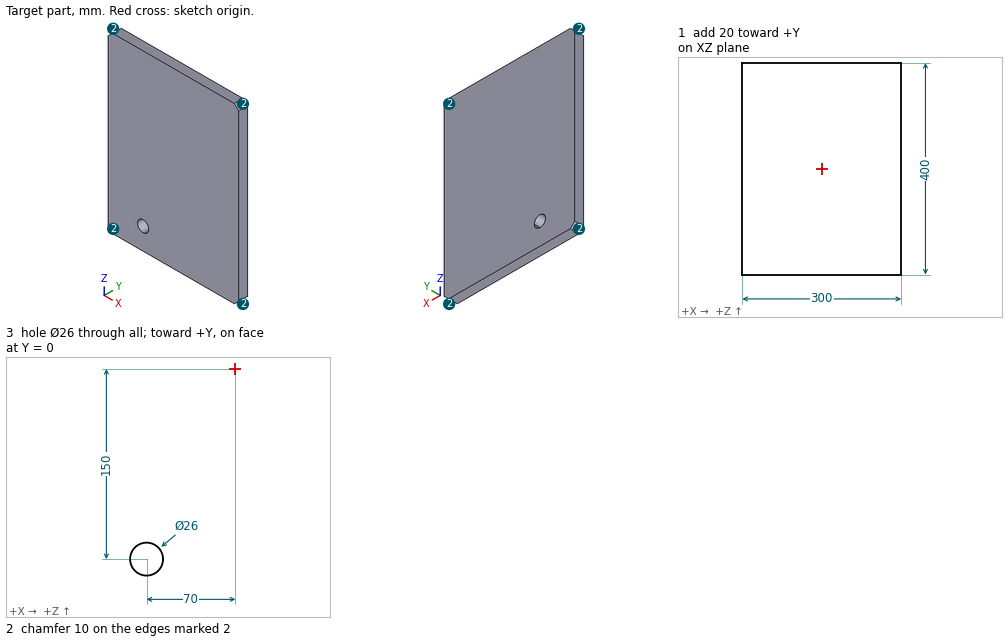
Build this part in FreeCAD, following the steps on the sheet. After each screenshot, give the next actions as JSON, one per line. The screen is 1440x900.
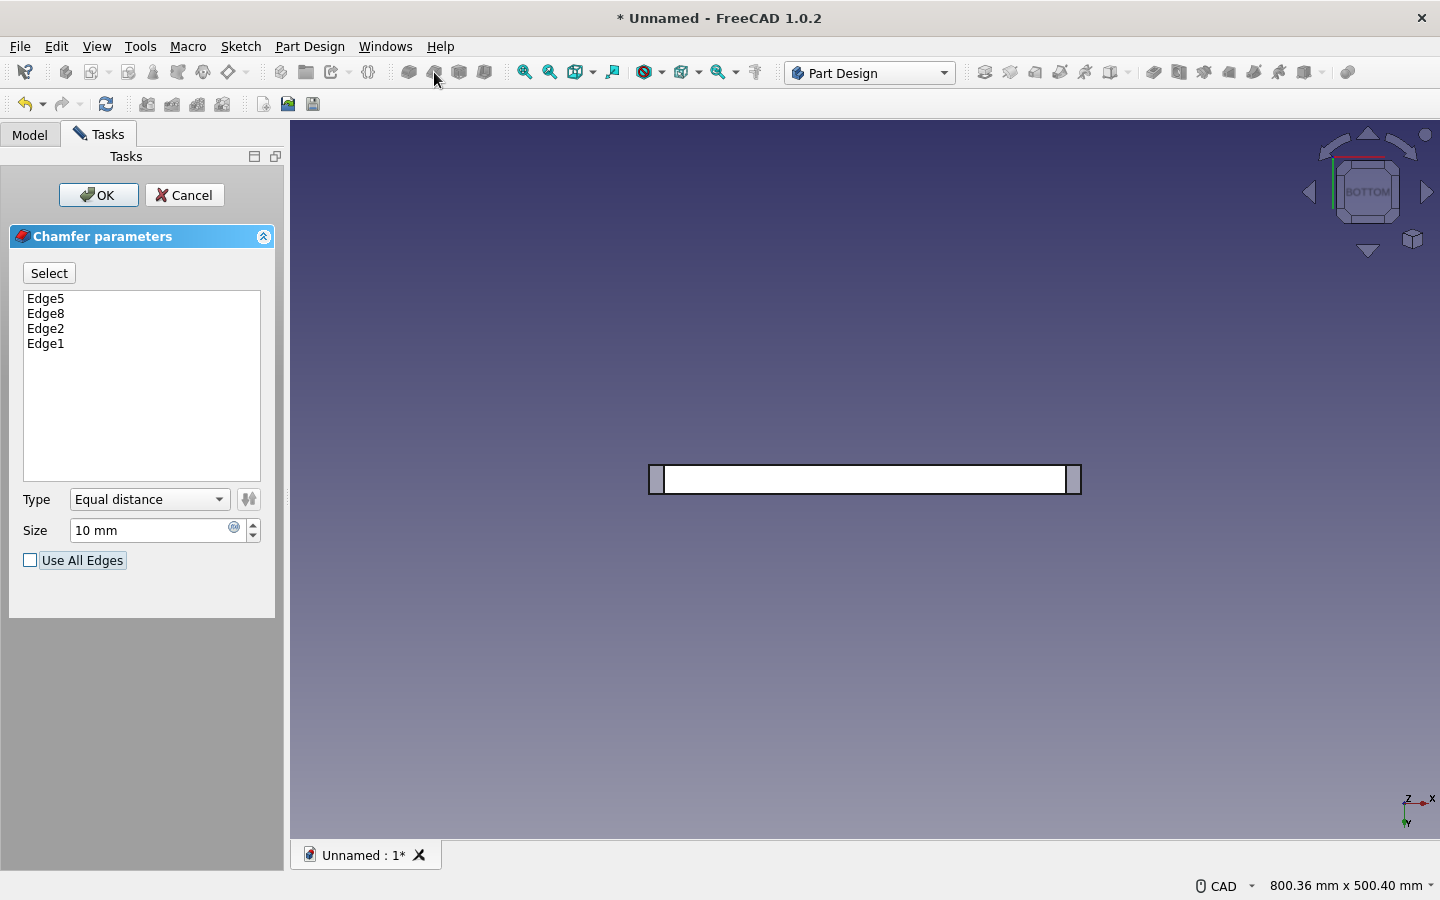
{"action": "left_click", "coordinate": [99, 195]}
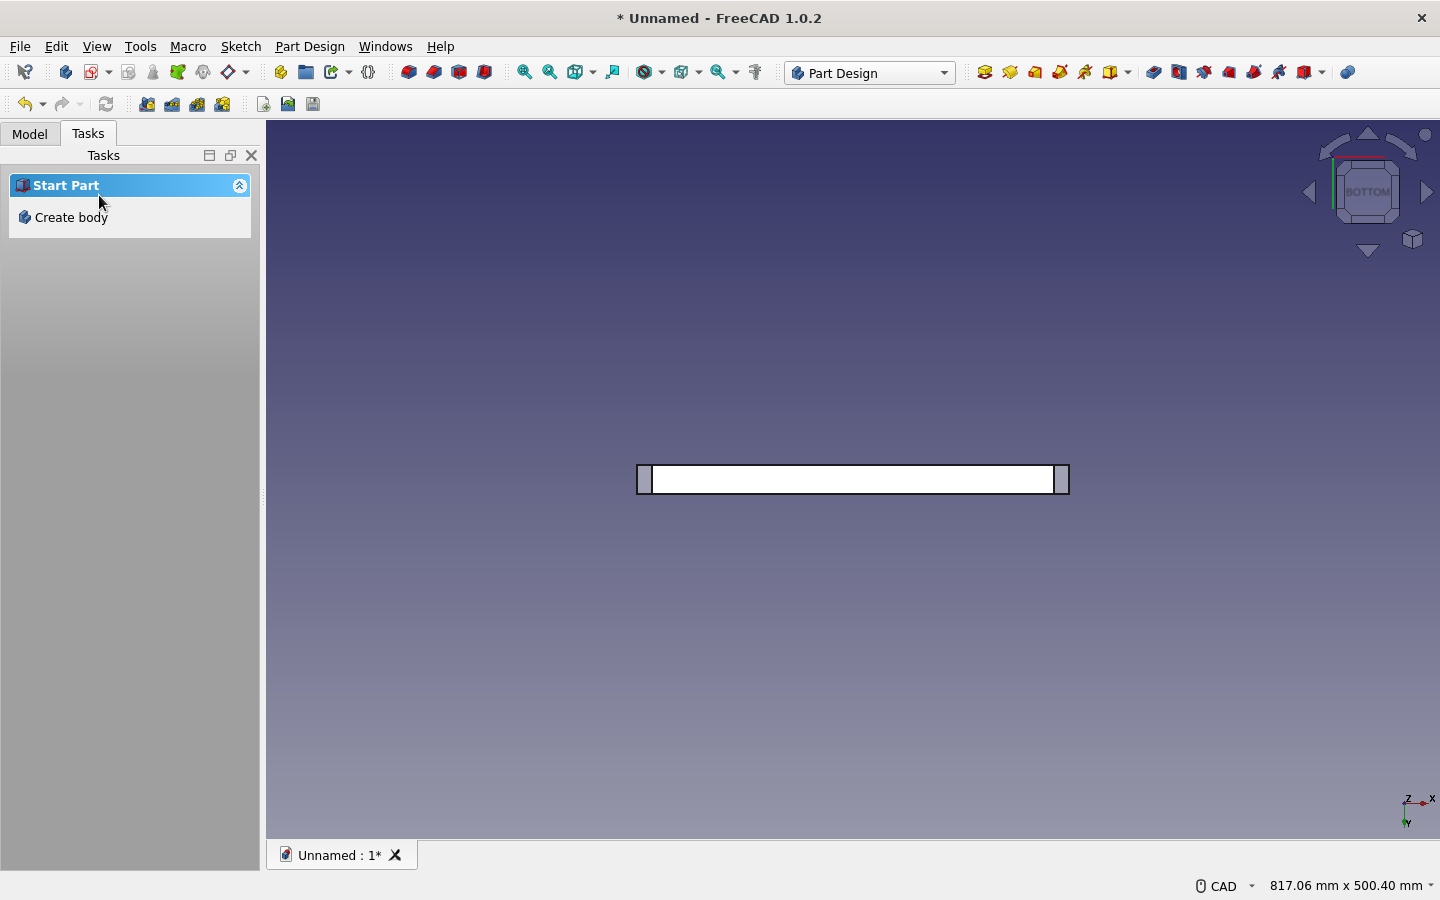
{"action": "left_click", "coordinate": [525, 72]}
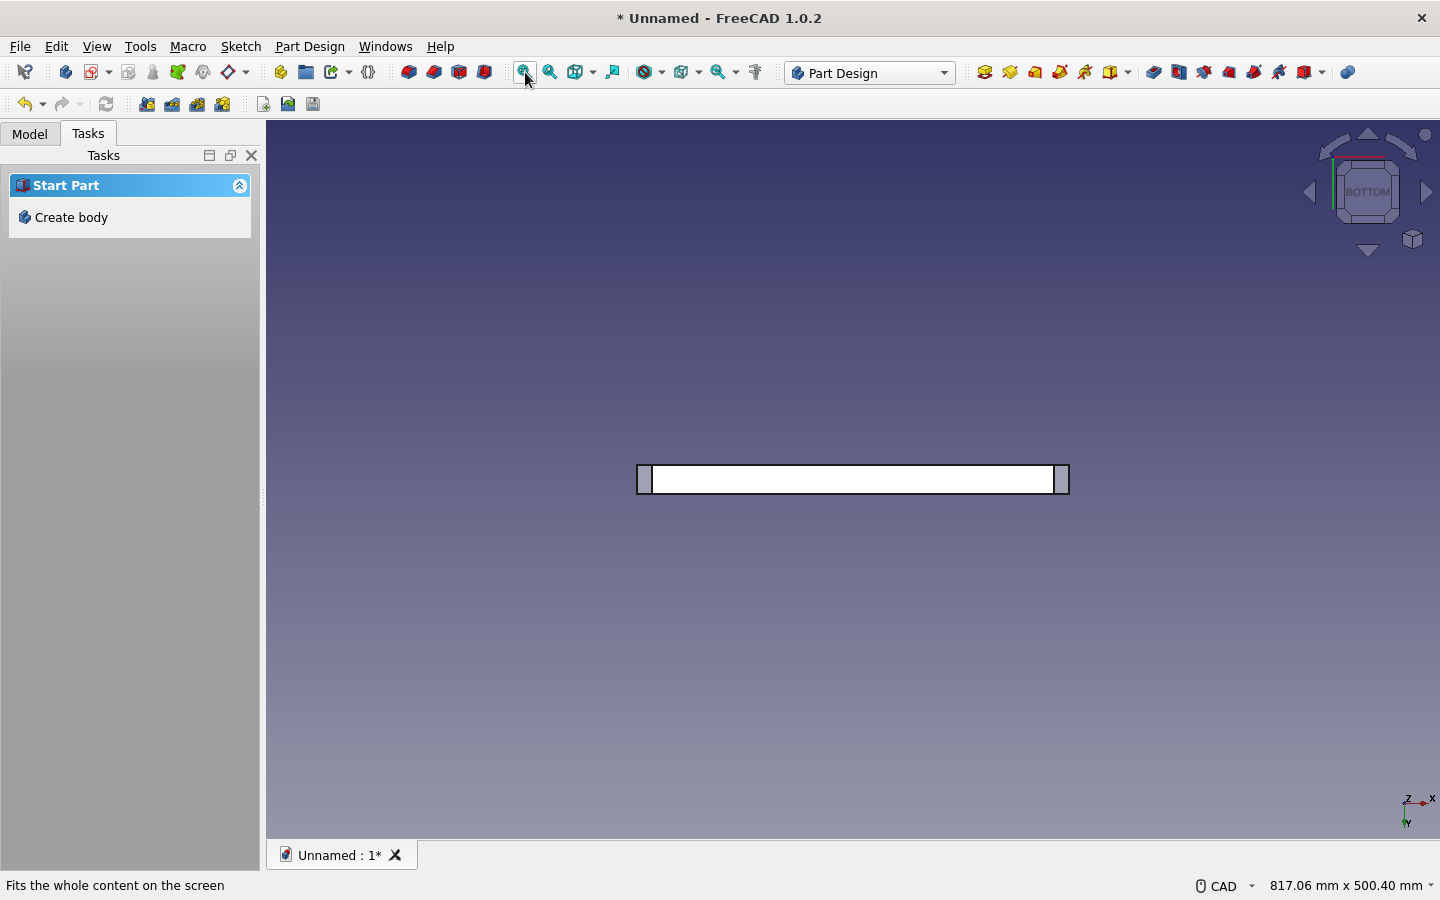
{"action": "key", "text": "0"}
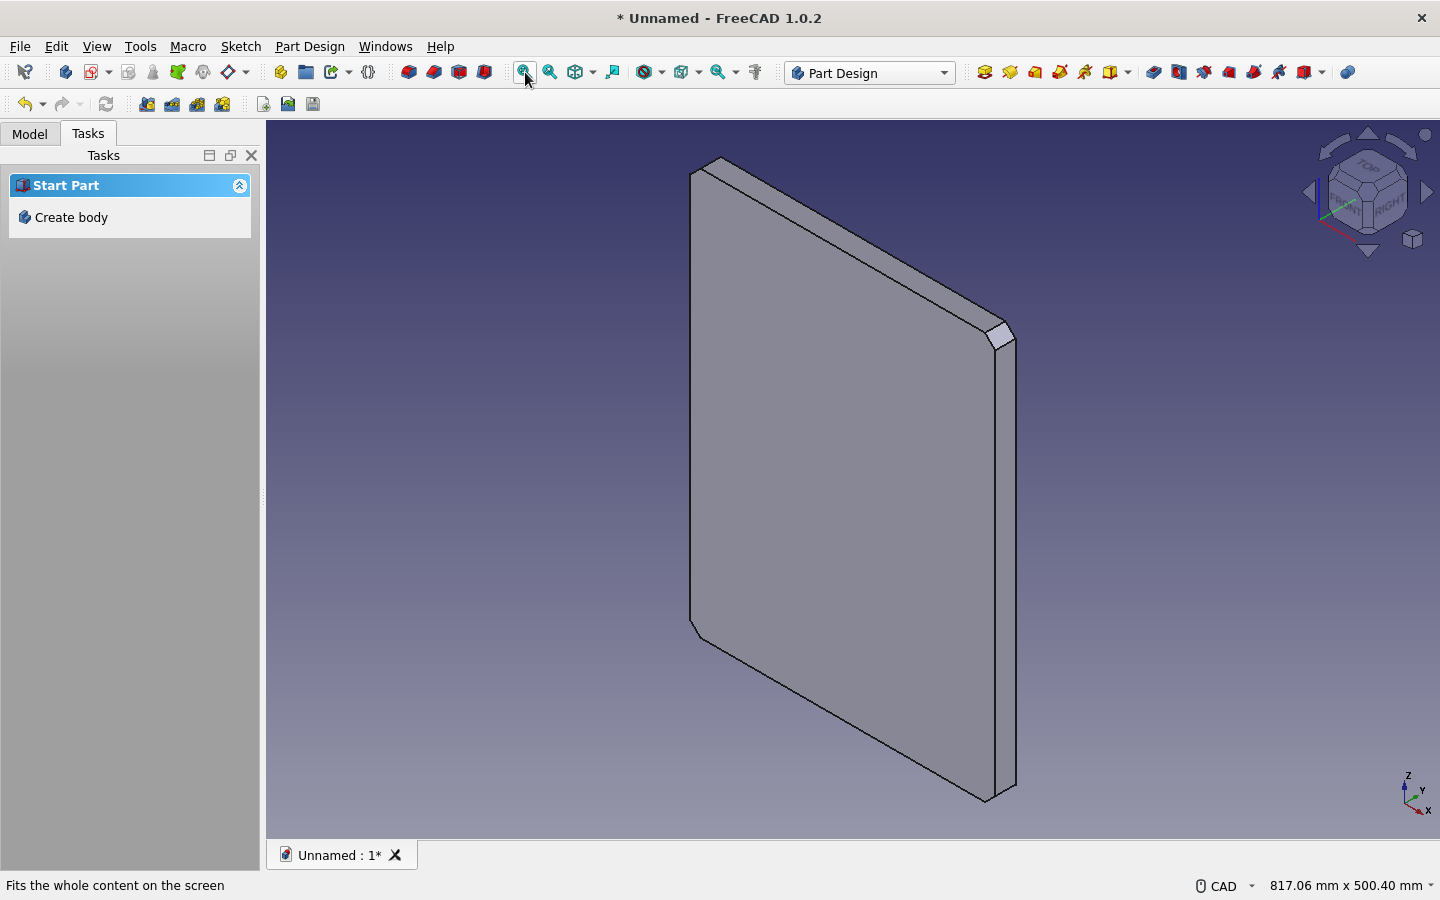
{"action": "left_click", "coordinate": [843, 484]}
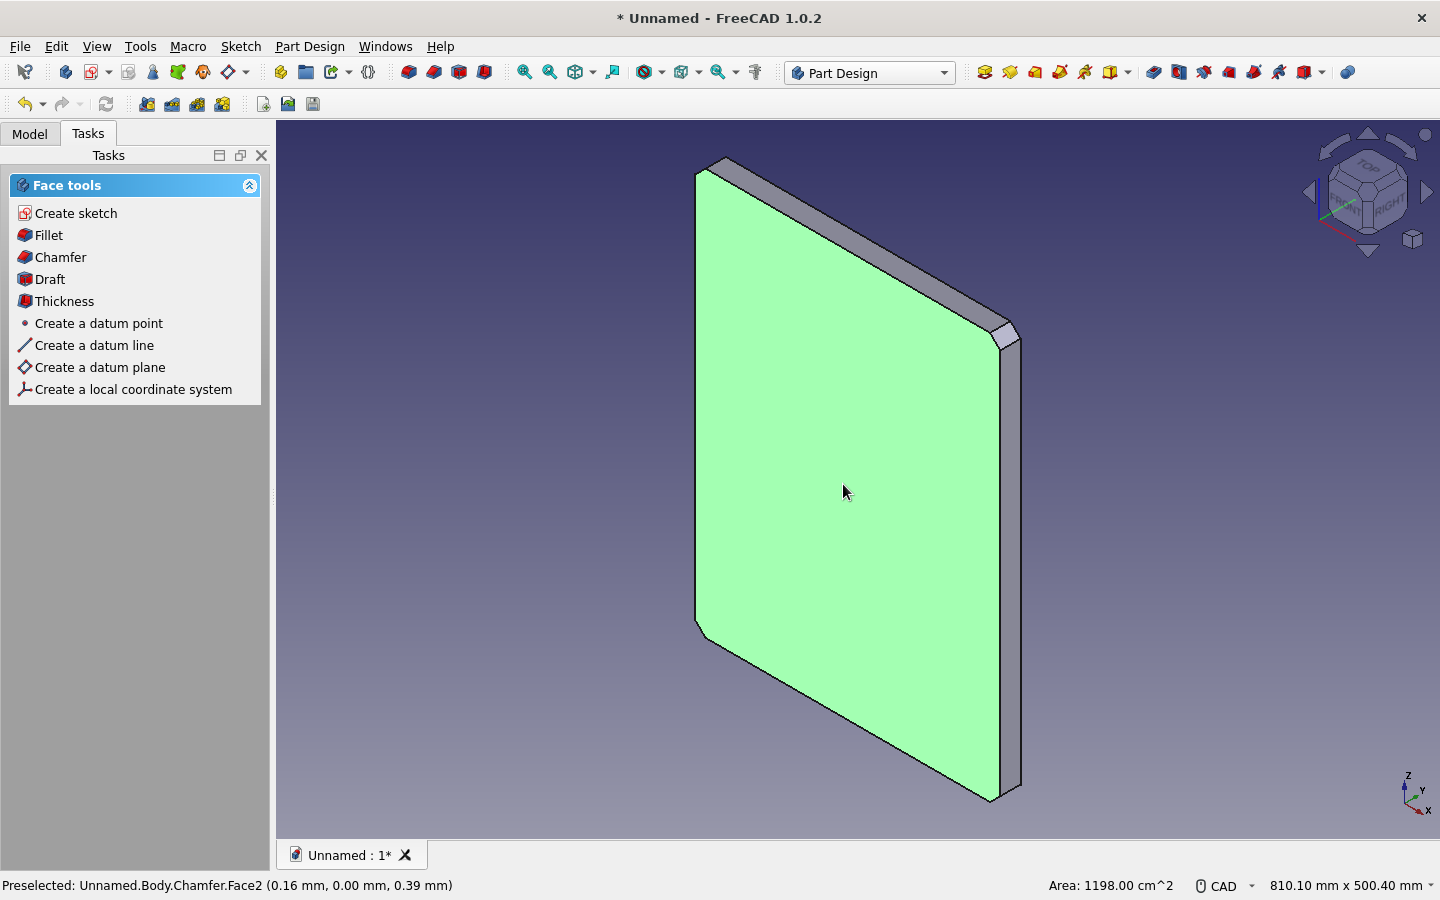
{"action": "left_click", "coordinate": [90, 72]}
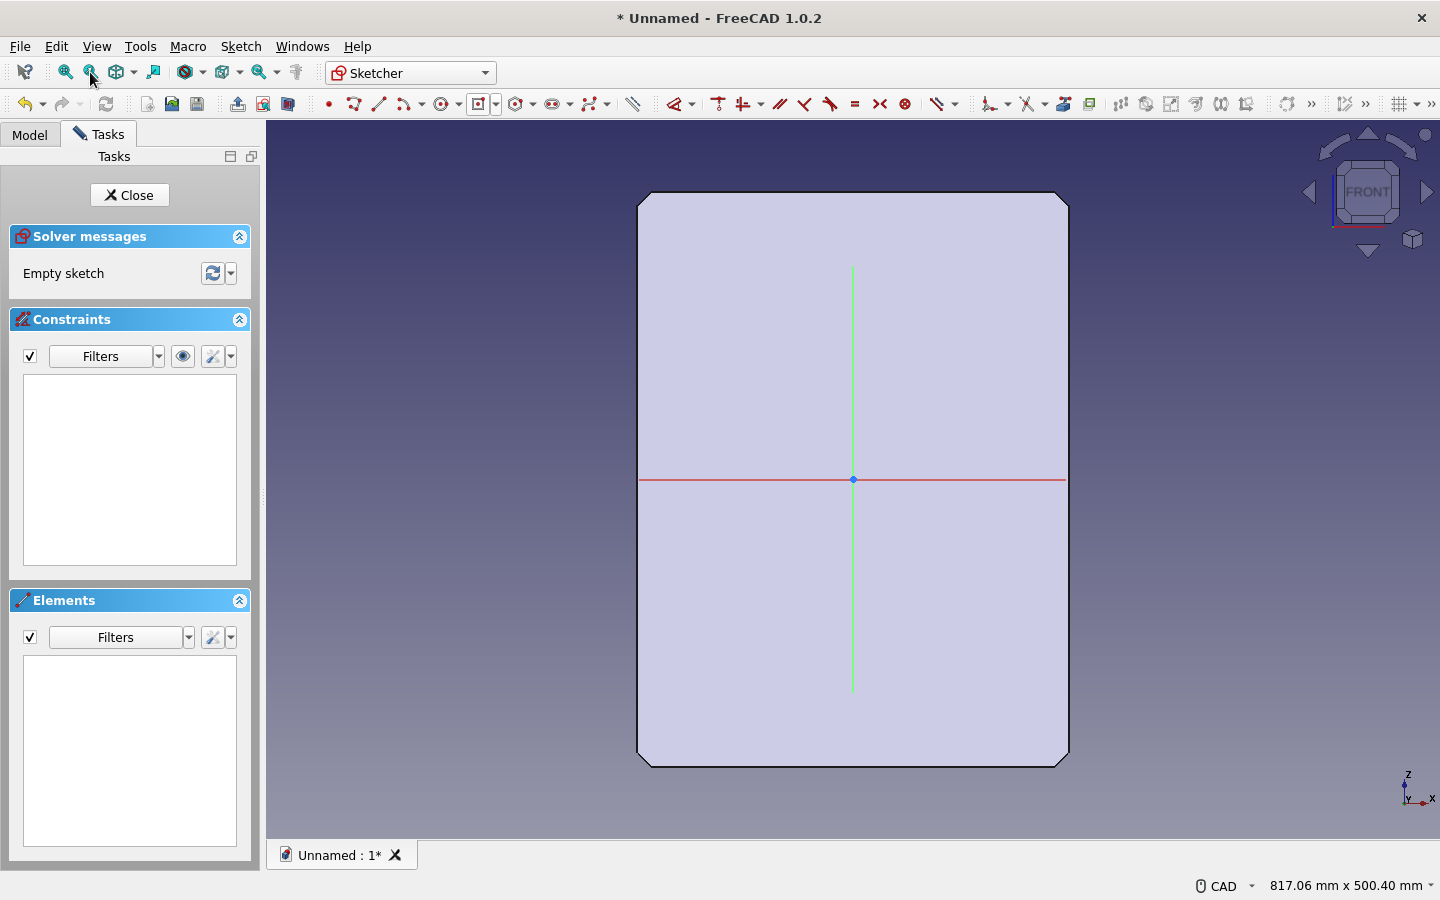
{"action": "scroll", "coordinate": [750, 712], "scroll_direction": "up", "scroll_amount": 13}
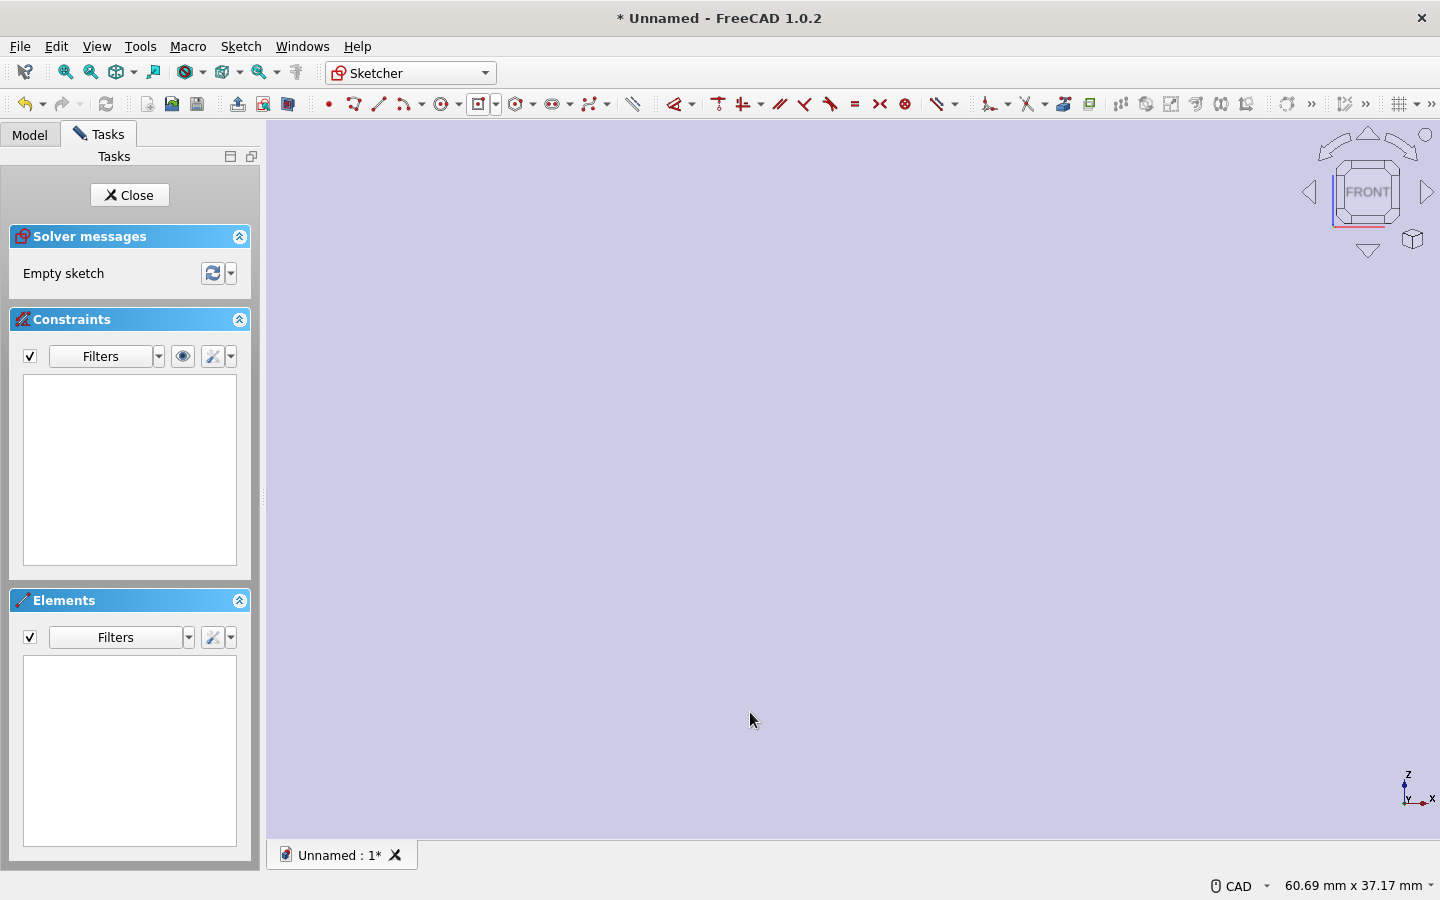
{"action": "left_click", "coordinate": [440, 104]}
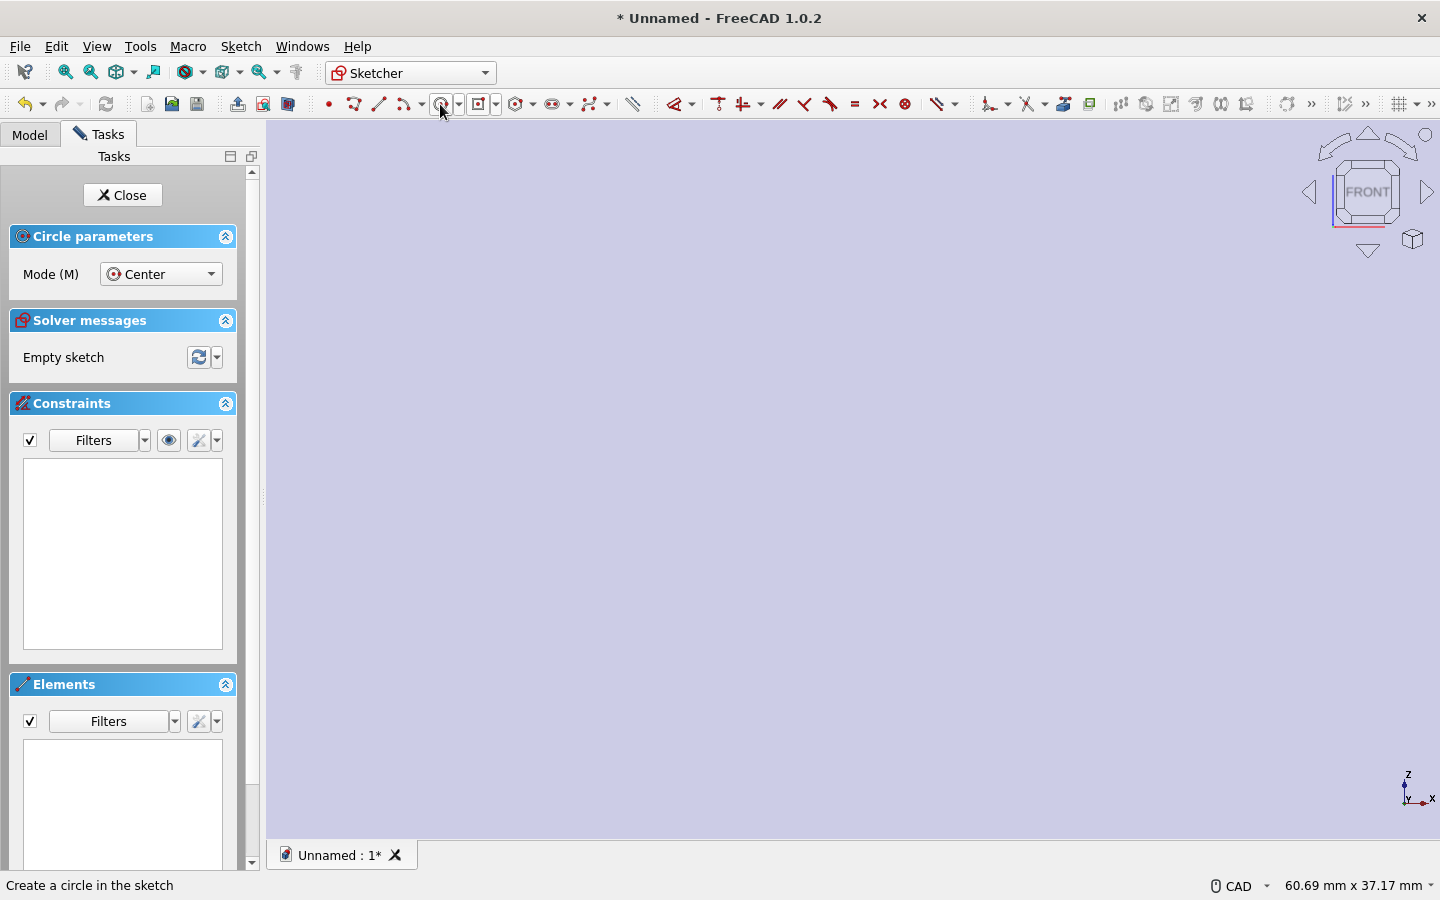
{"action": "left_click", "coordinate": [777, 473]}
{"action": "left_click", "coordinate": [955, 295]}
{"action": "key", "text": "Escape"}